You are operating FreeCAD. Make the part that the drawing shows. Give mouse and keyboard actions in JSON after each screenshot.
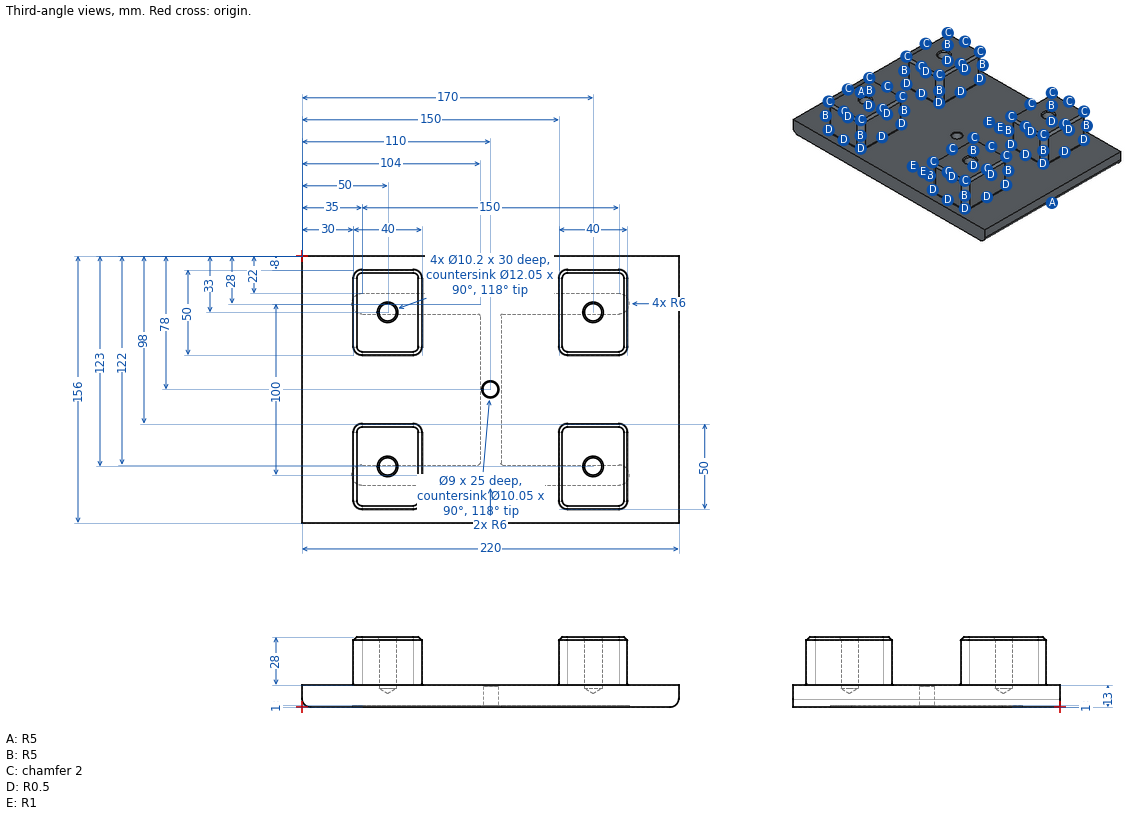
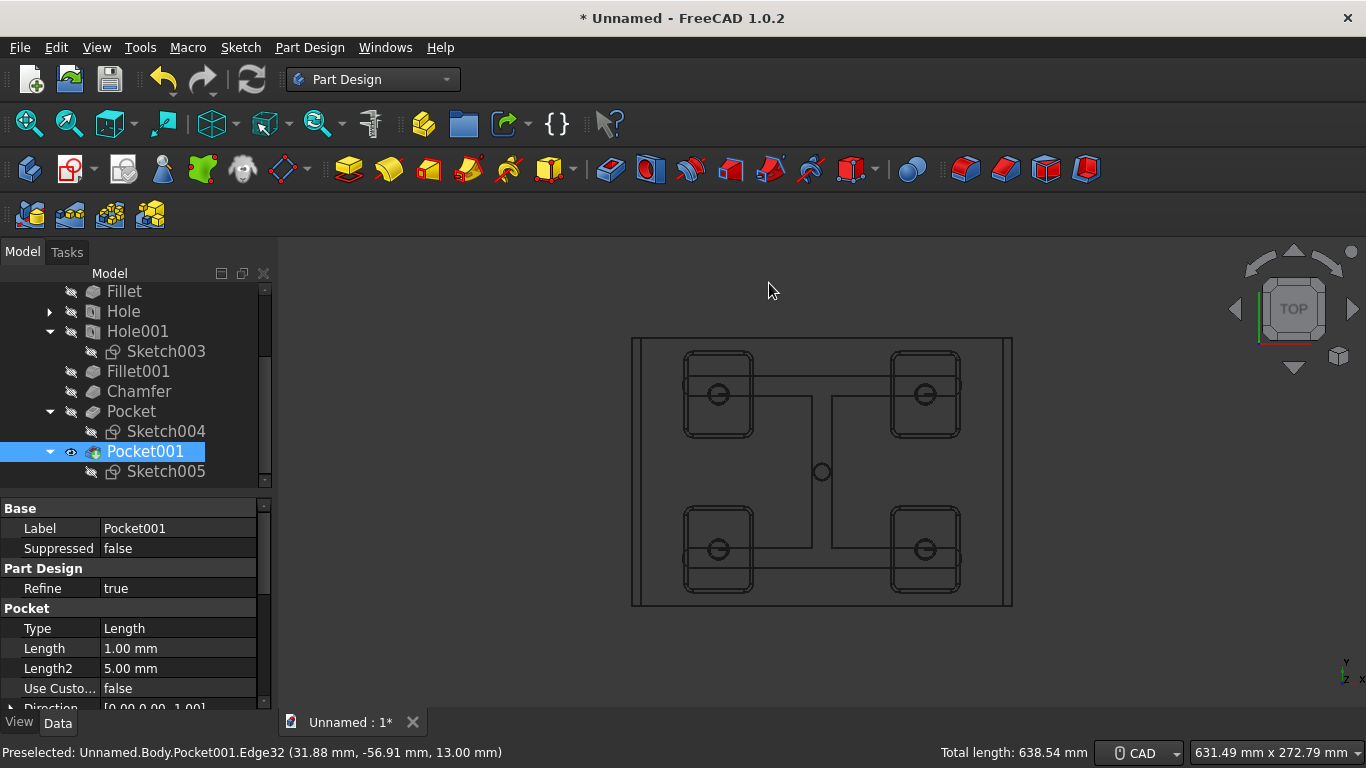
{"action": "scroll", "coordinate": [893, 589], "scroll_direction": "up", "scroll_amount": 6}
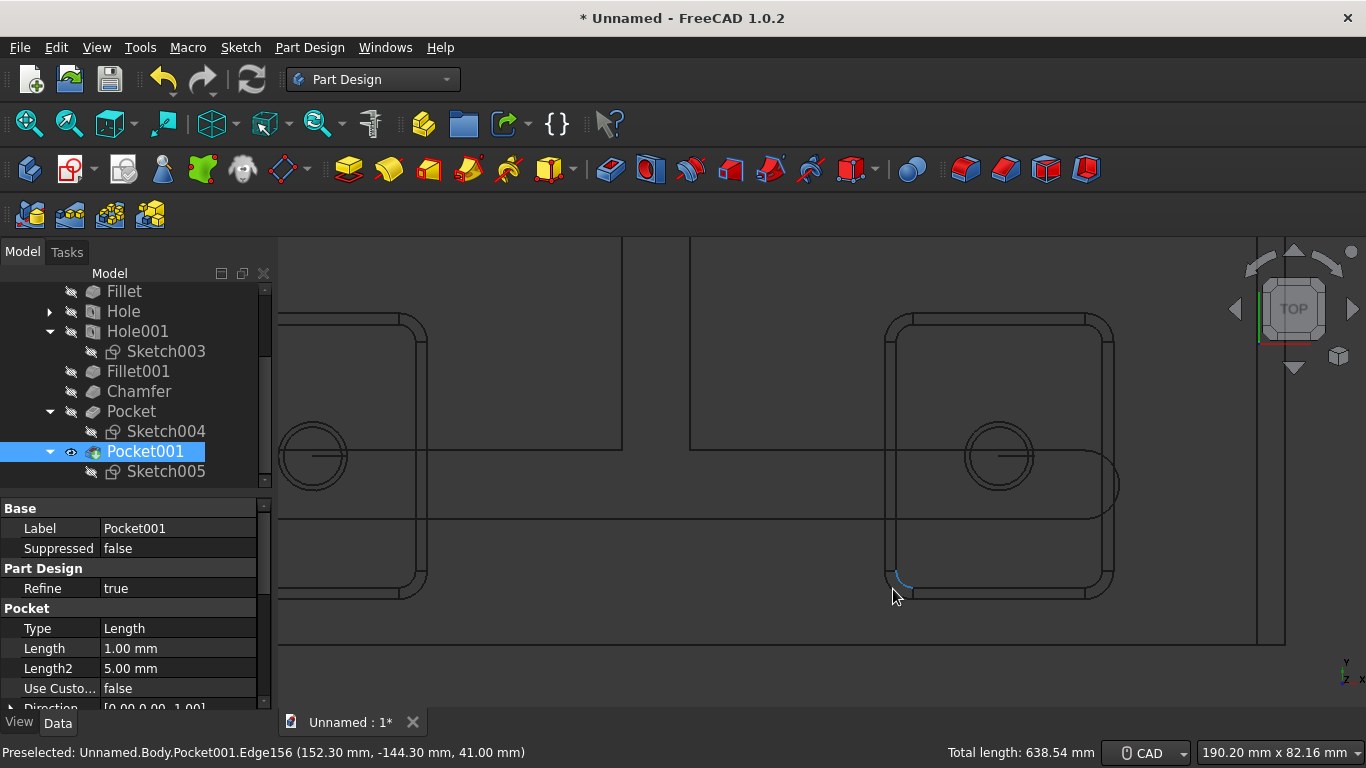
{"action": "left_click", "coordinate": [30, 124]}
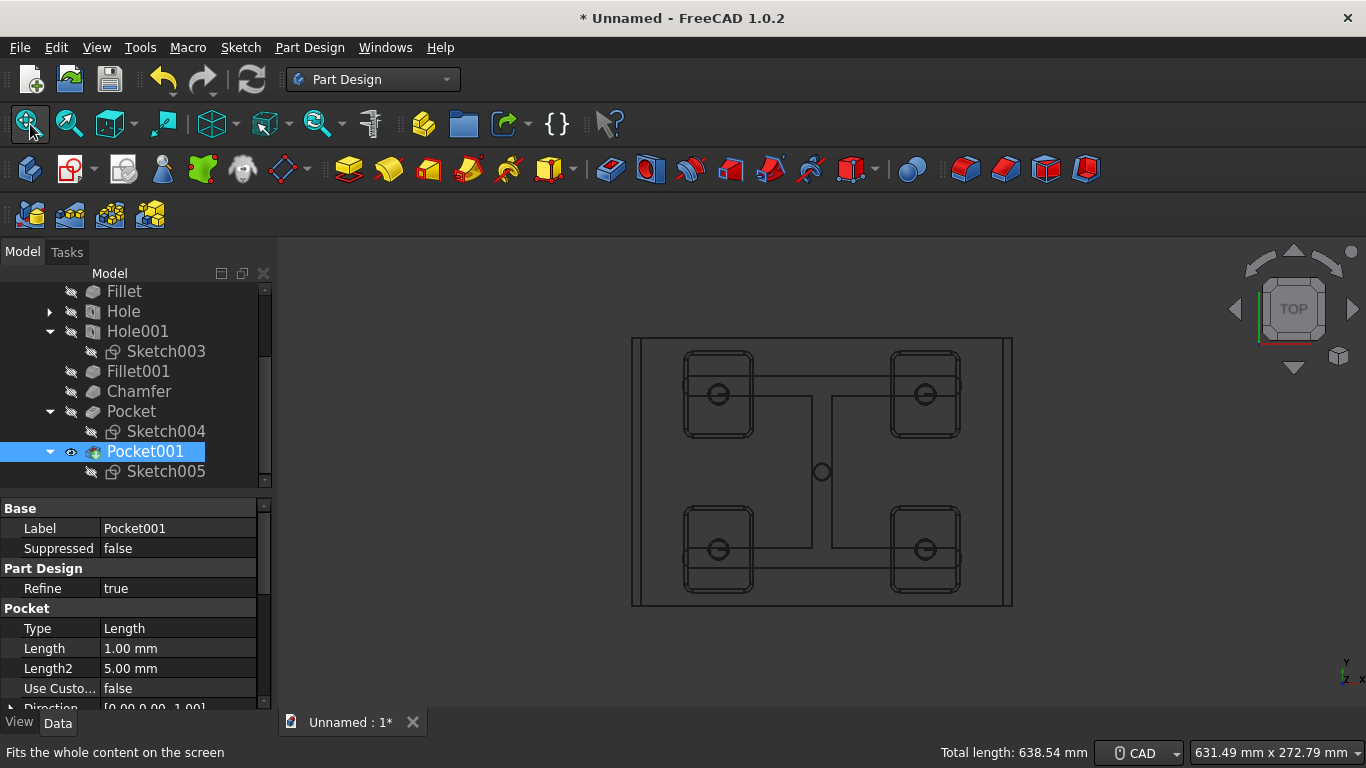
{"action": "key", "text": "1"}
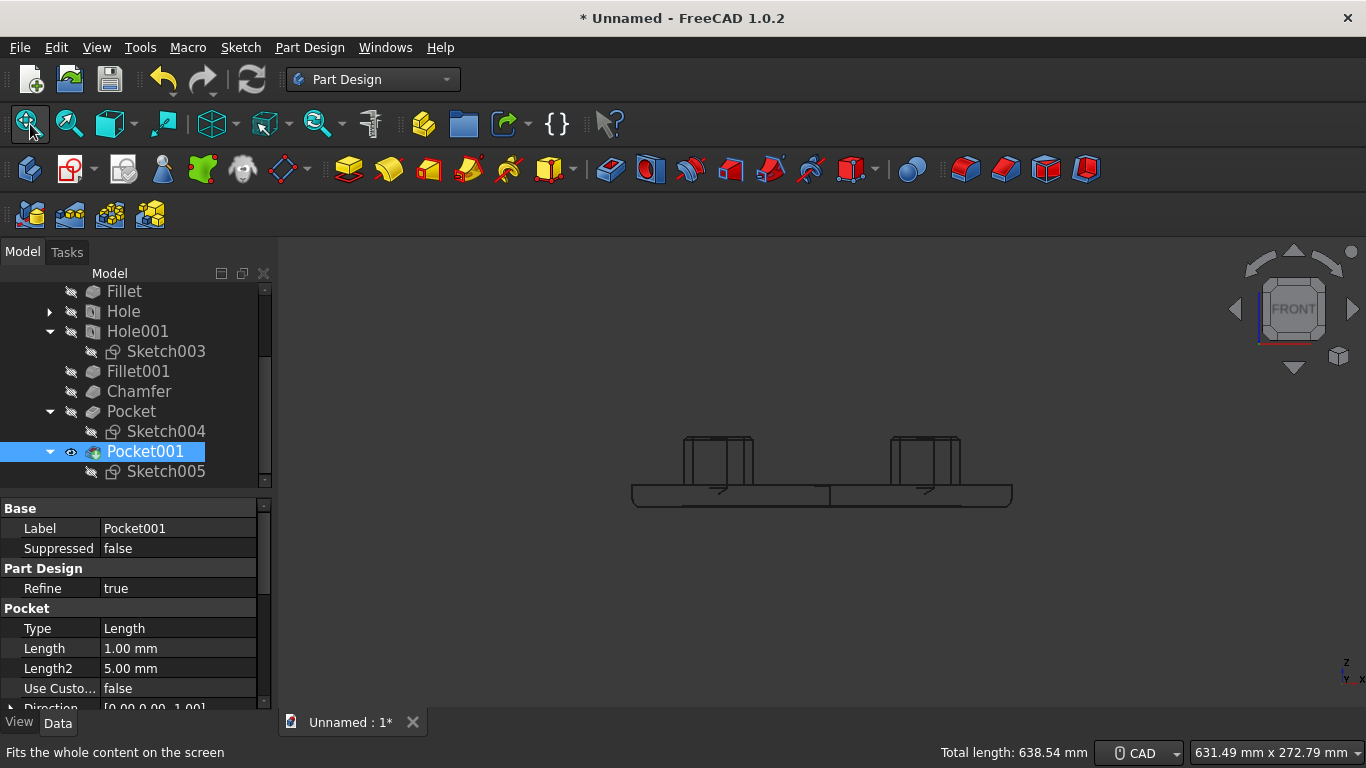
{"action": "left_click", "coordinate": [30, 124]}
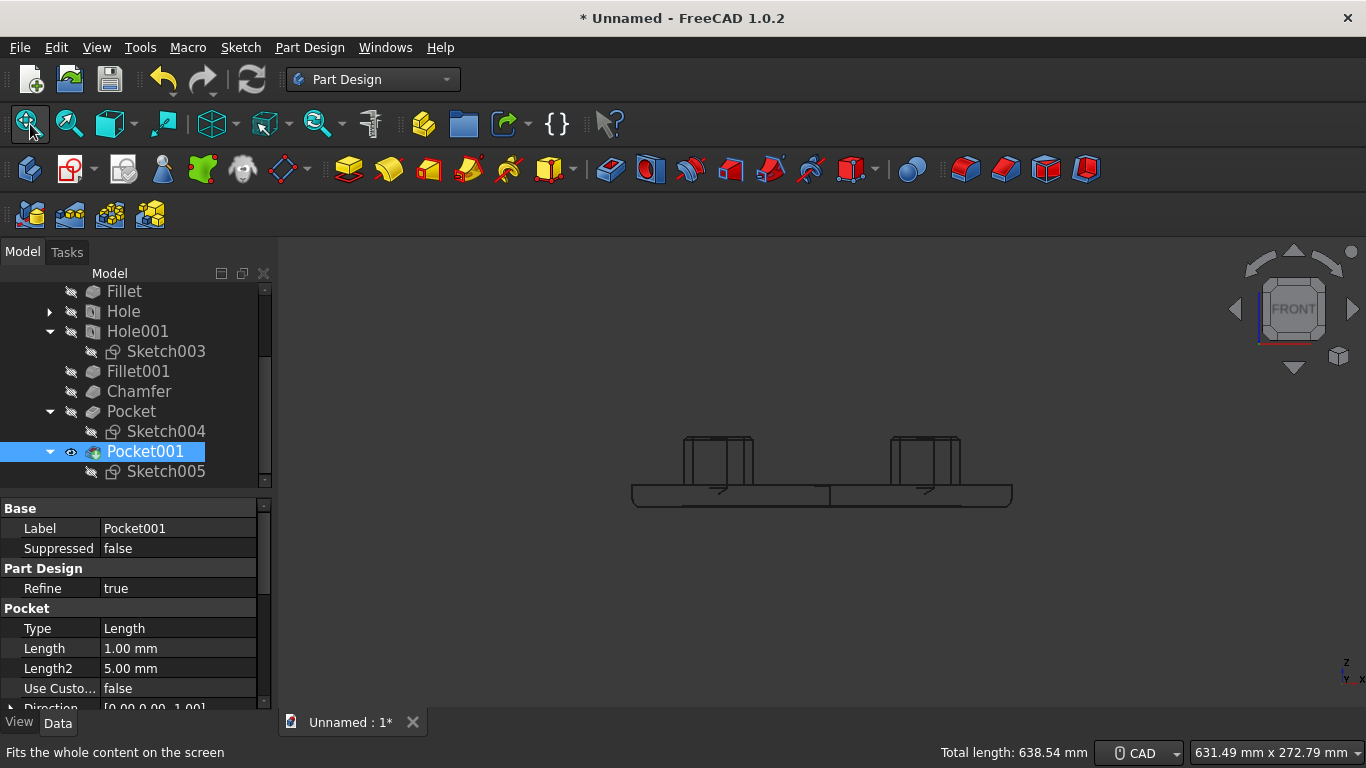
{"action": "scroll", "coordinate": [893, 484], "scroll_direction": "up", "scroll_amount": 6}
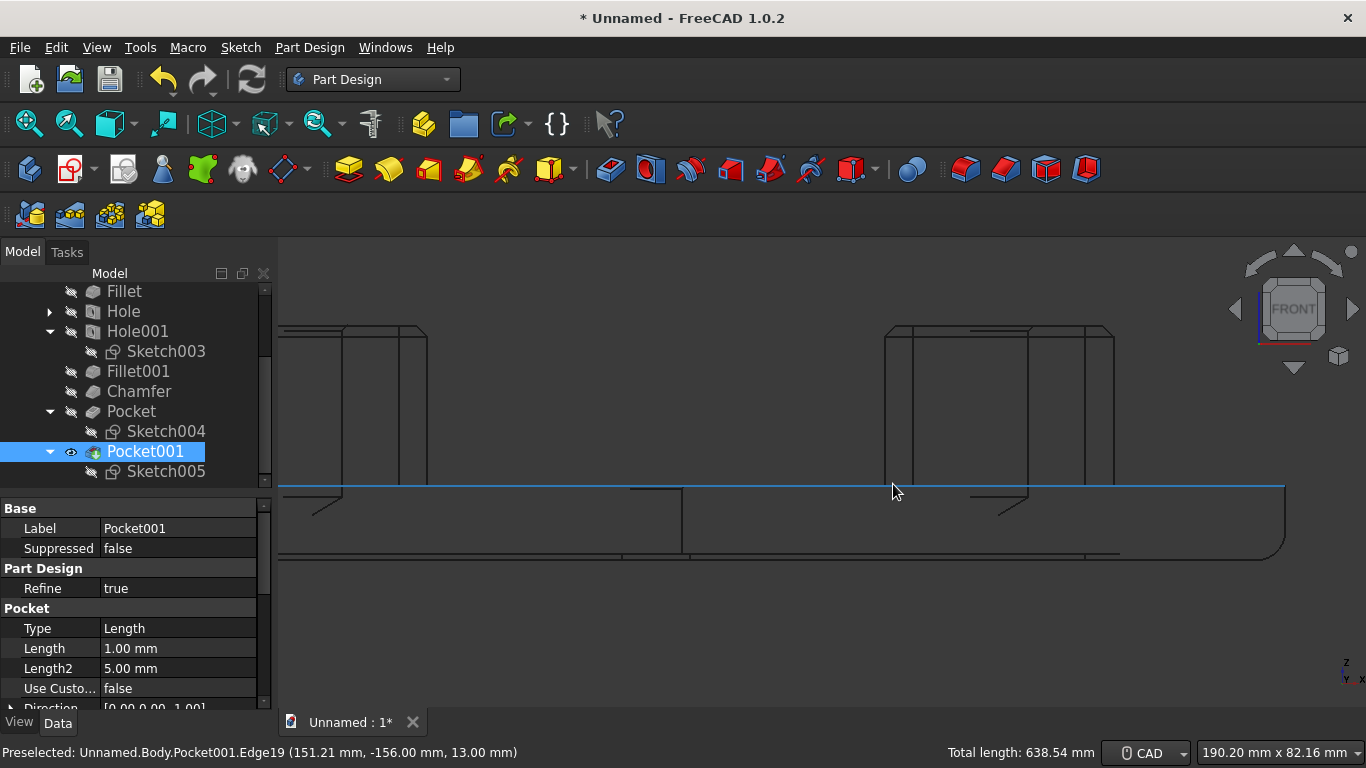
{"action": "left_click", "coordinate": [30, 124]}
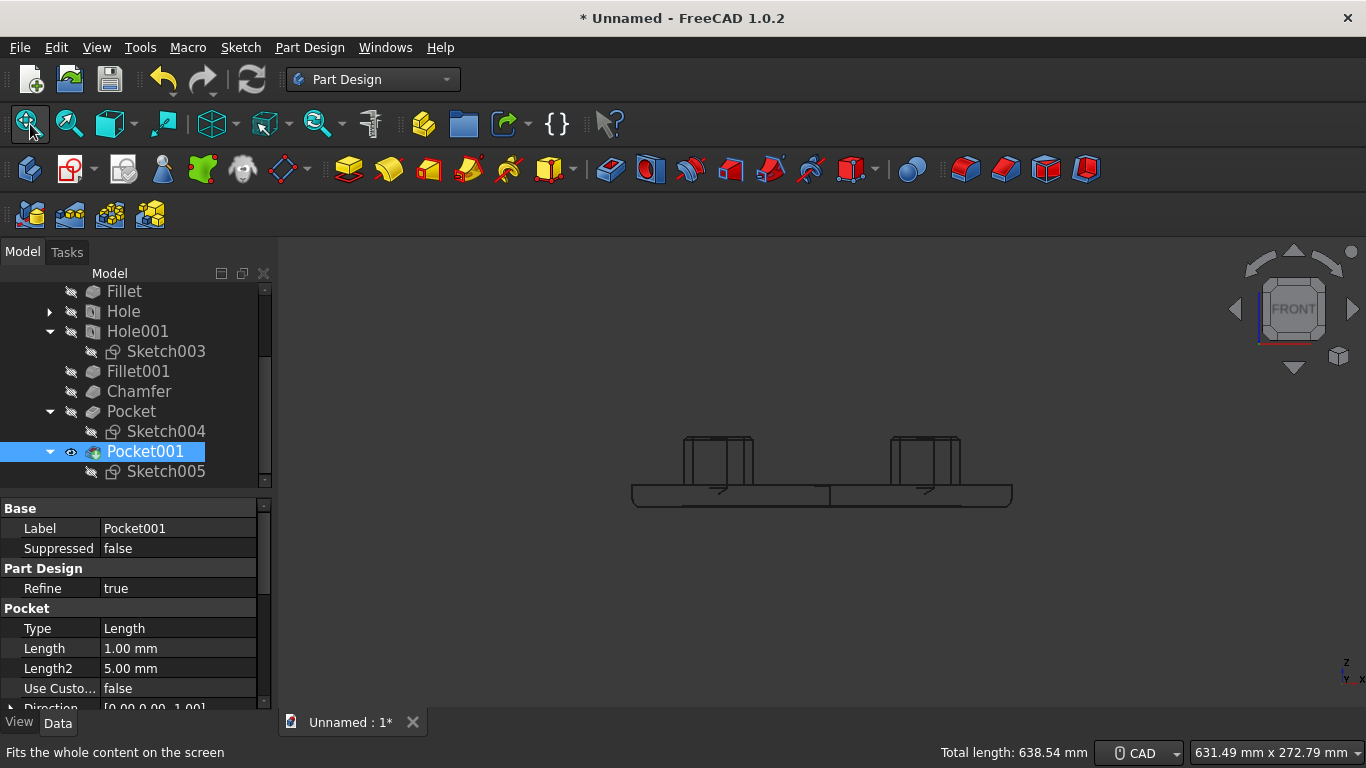
{"action": "key", "text": "3"}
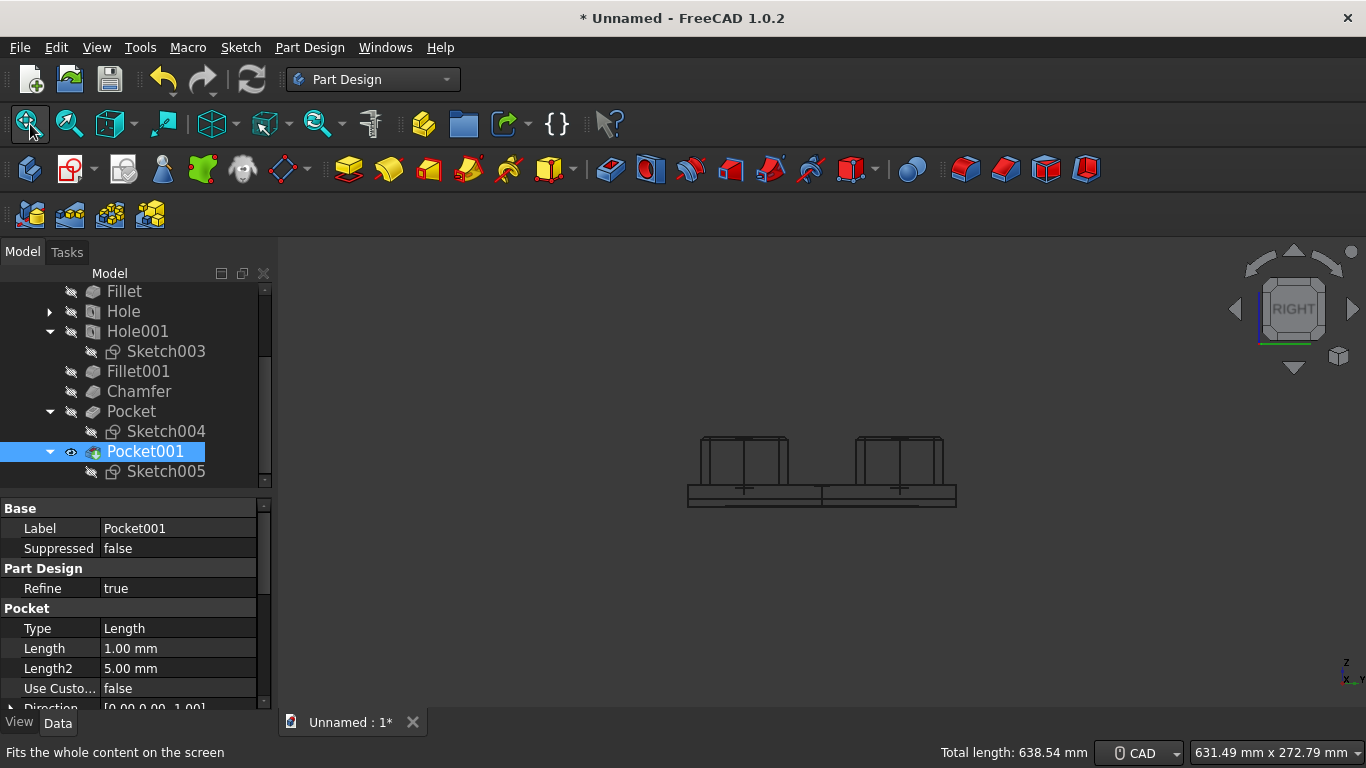
{"action": "key", "text": "v f"}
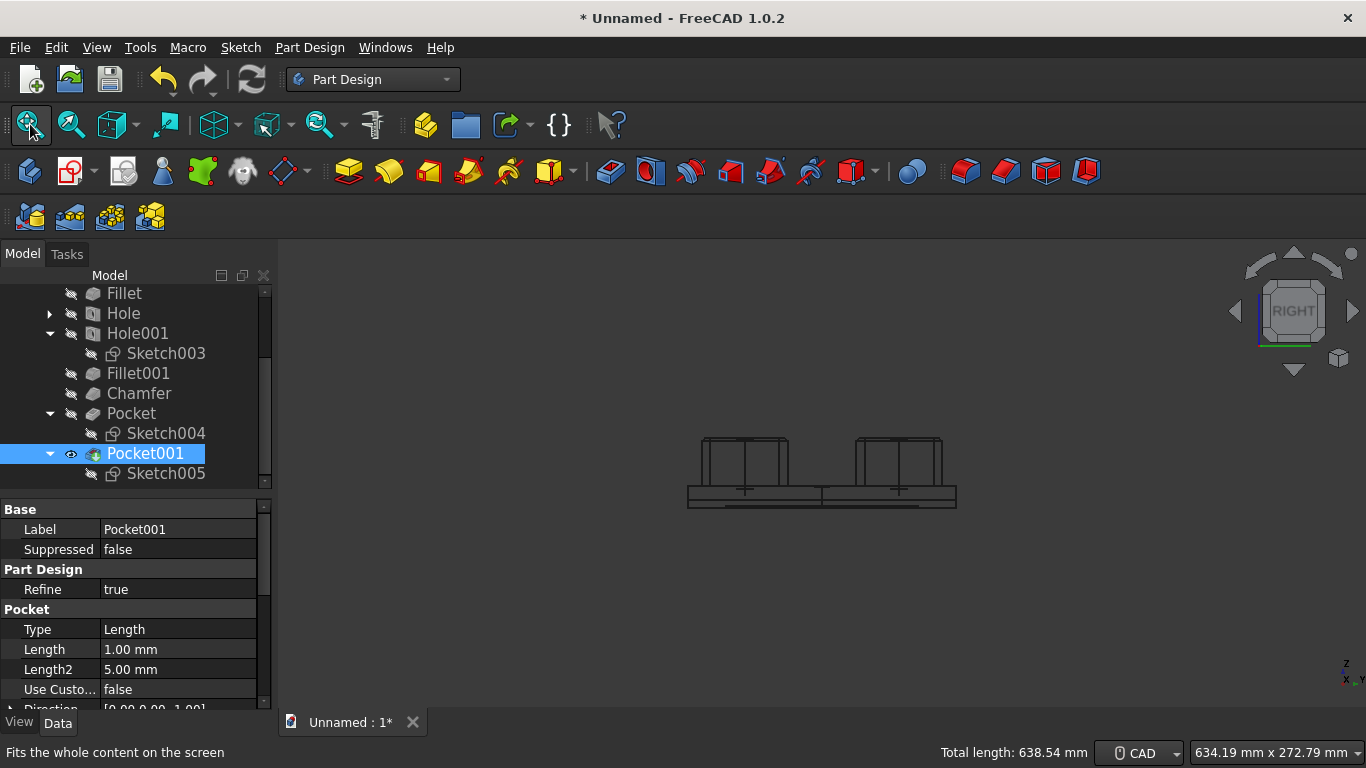
{"action": "scroll", "coordinate": [704, 485], "scroll_direction": "up", "scroll_amount": 6}